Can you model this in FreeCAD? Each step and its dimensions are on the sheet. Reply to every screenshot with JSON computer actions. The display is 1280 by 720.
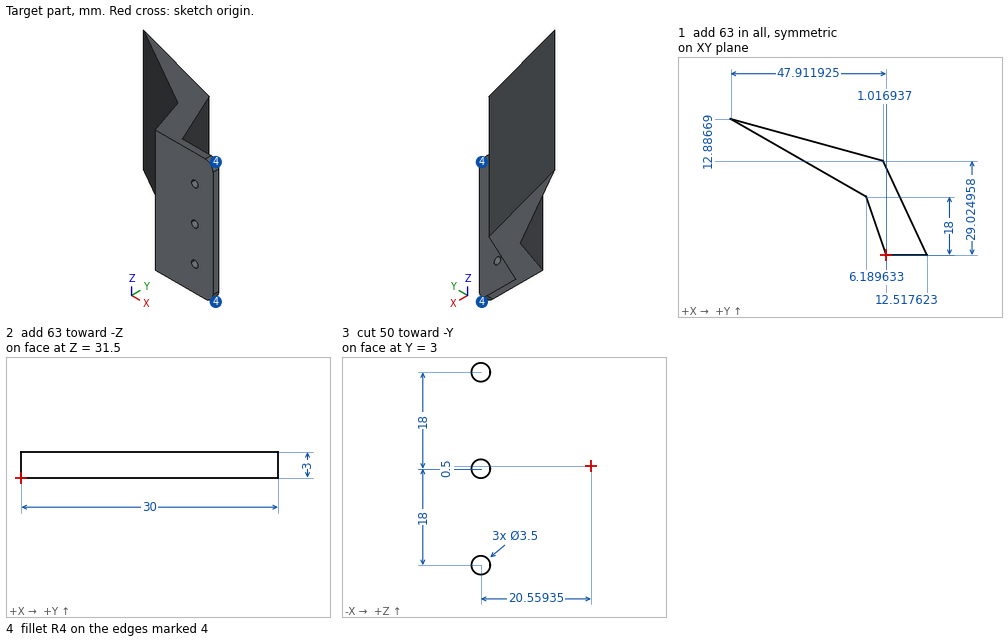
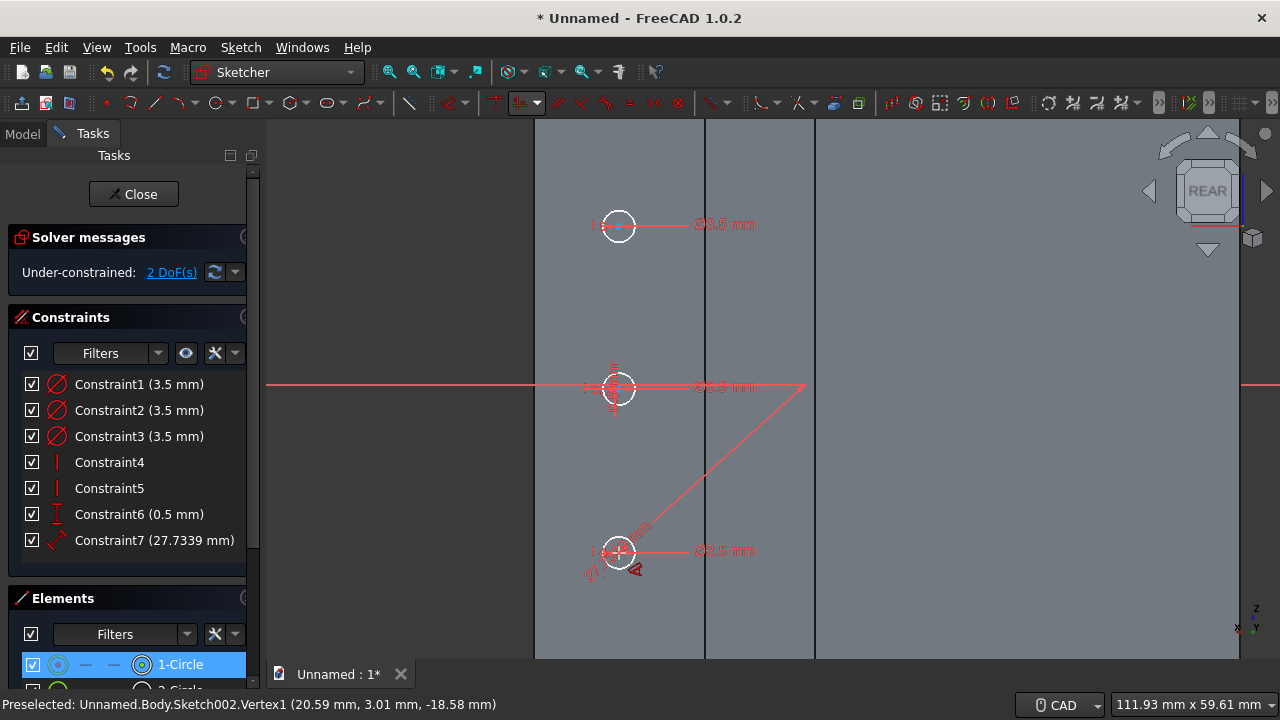
{"action": "left_click", "coordinate": [619, 389]}
{"action": "left_click", "coordinate": [585, 471]}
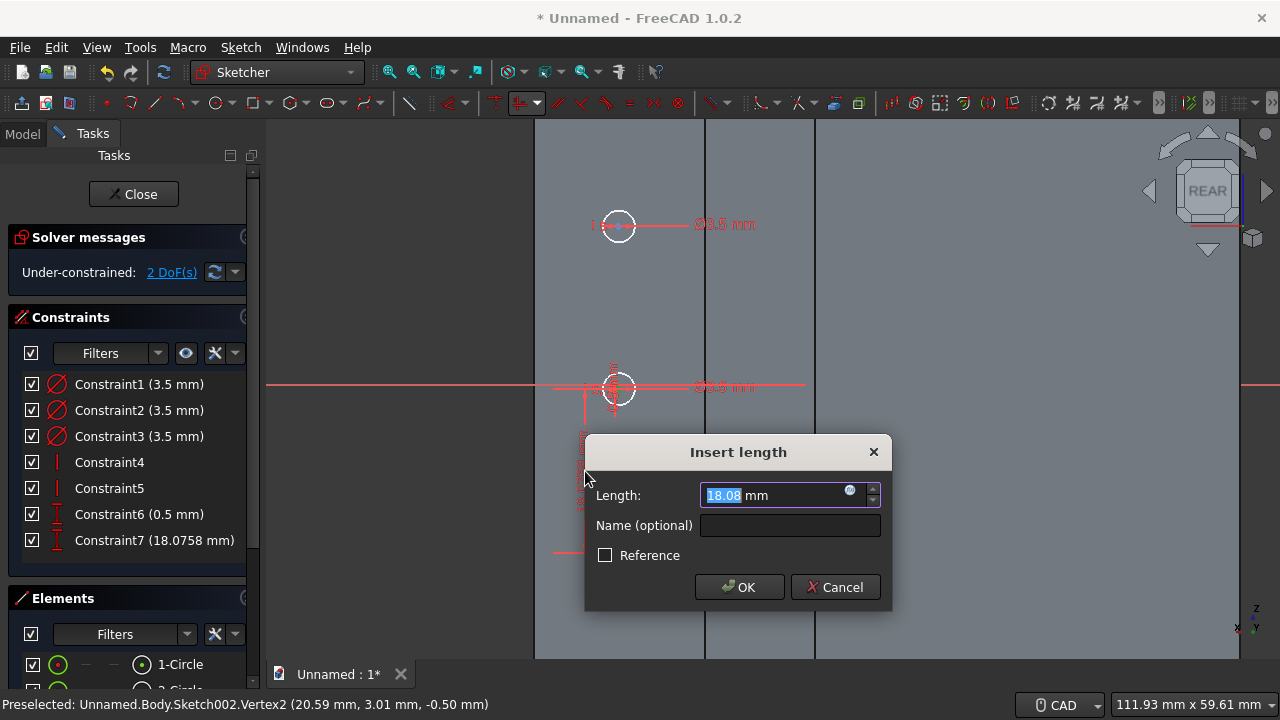
{"action": "type", "text": "18"}
{"action": "key", "text": "Return"}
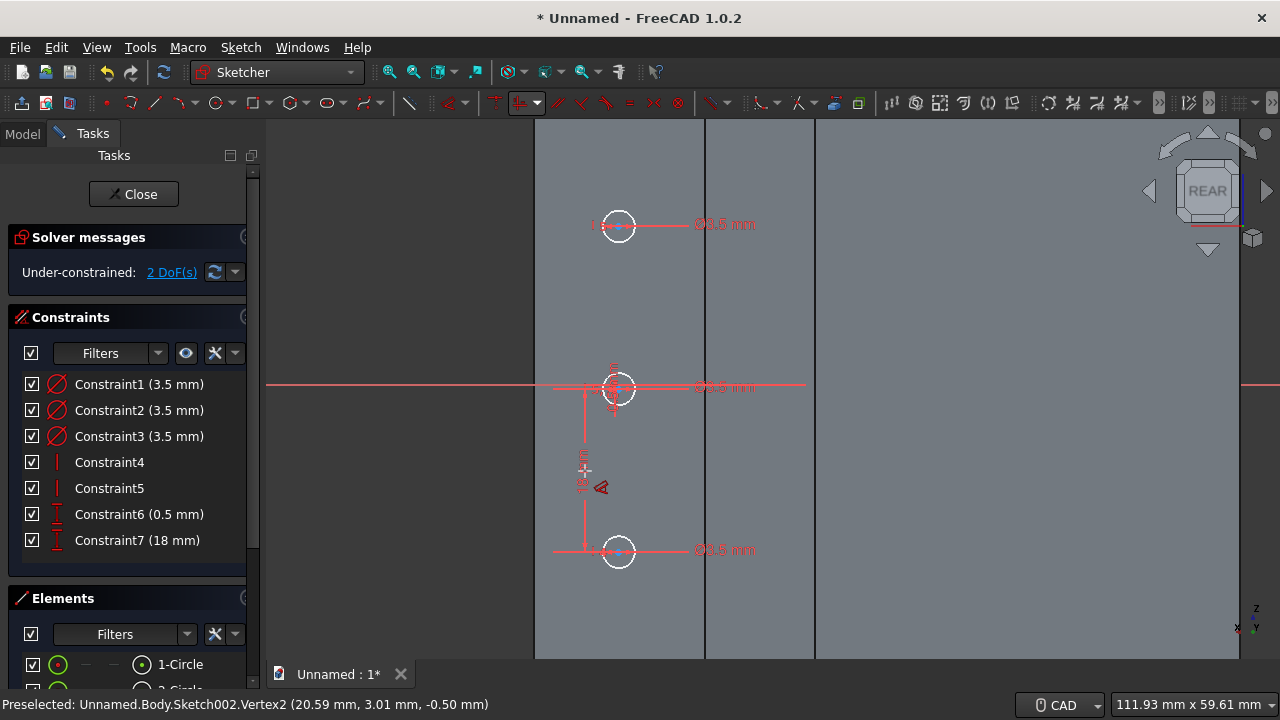
{"action": "left_click", "coordinate": [619, 389]}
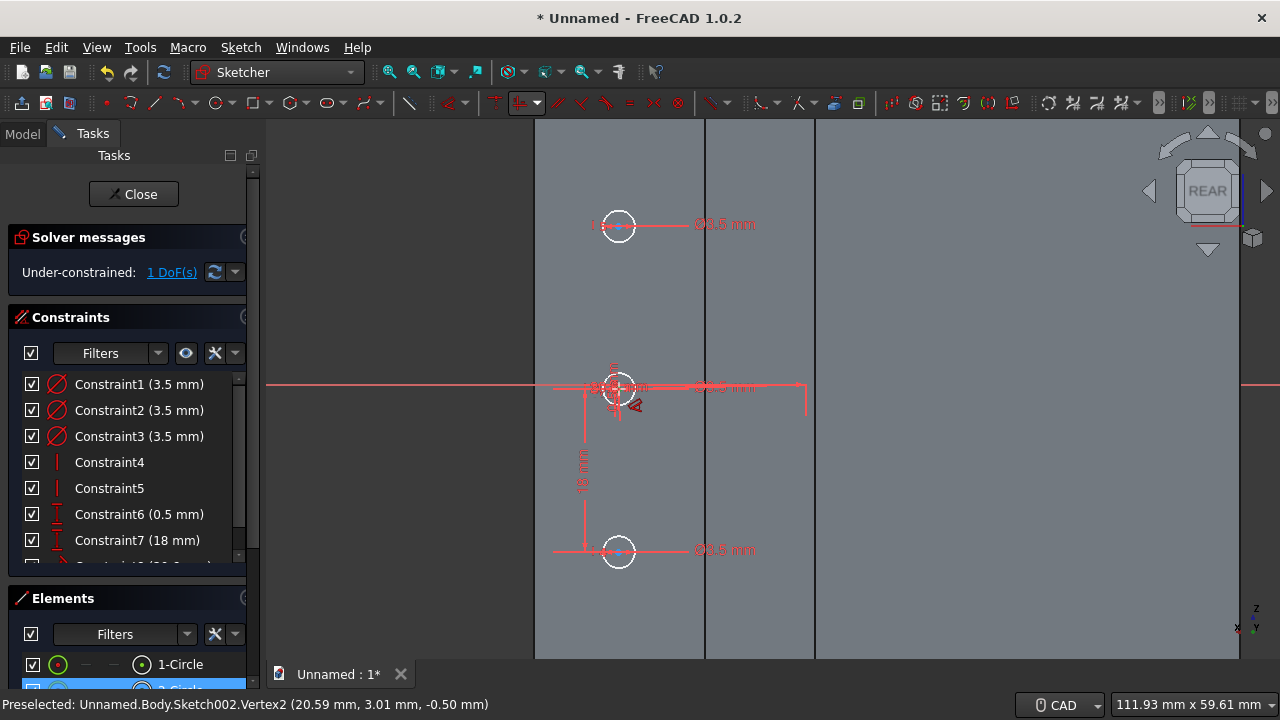
{"action": "left_click", "coordinate": [619, 226]}
{"action": "left_click", "coordinate": [585, 308]}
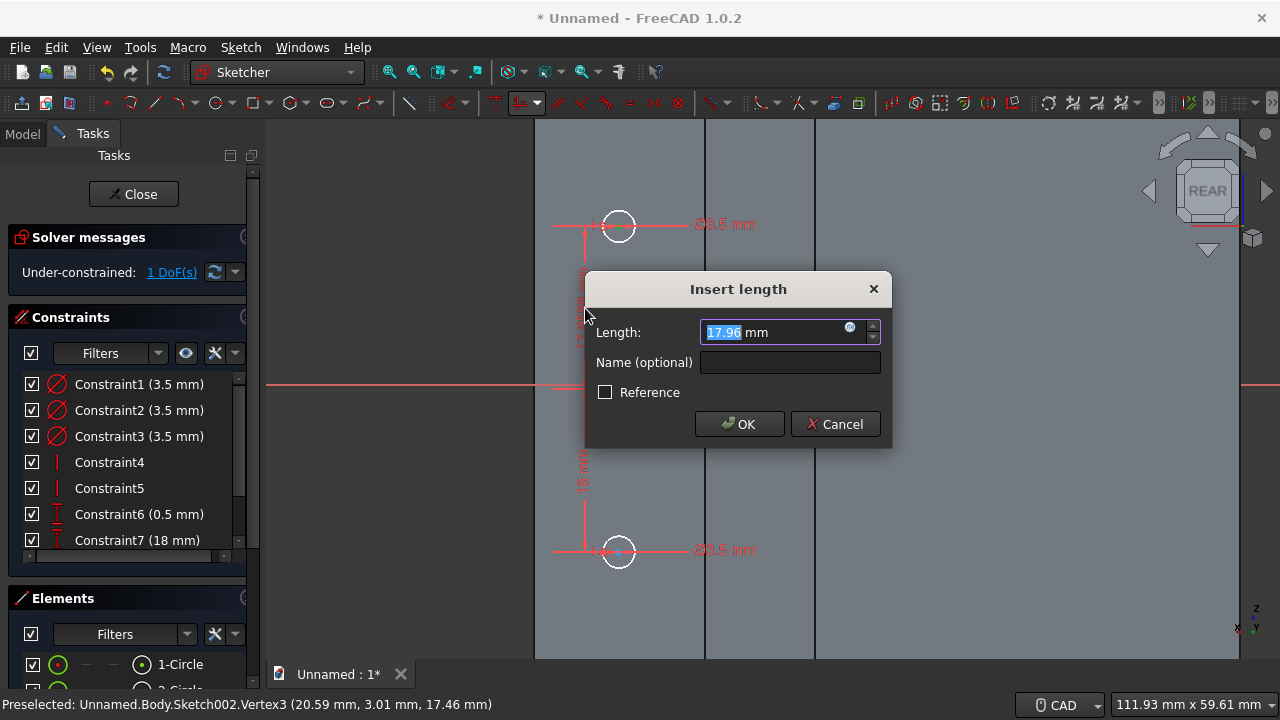
{"action": "type", "text": "18"}
{"action": "key", "text": "Return"}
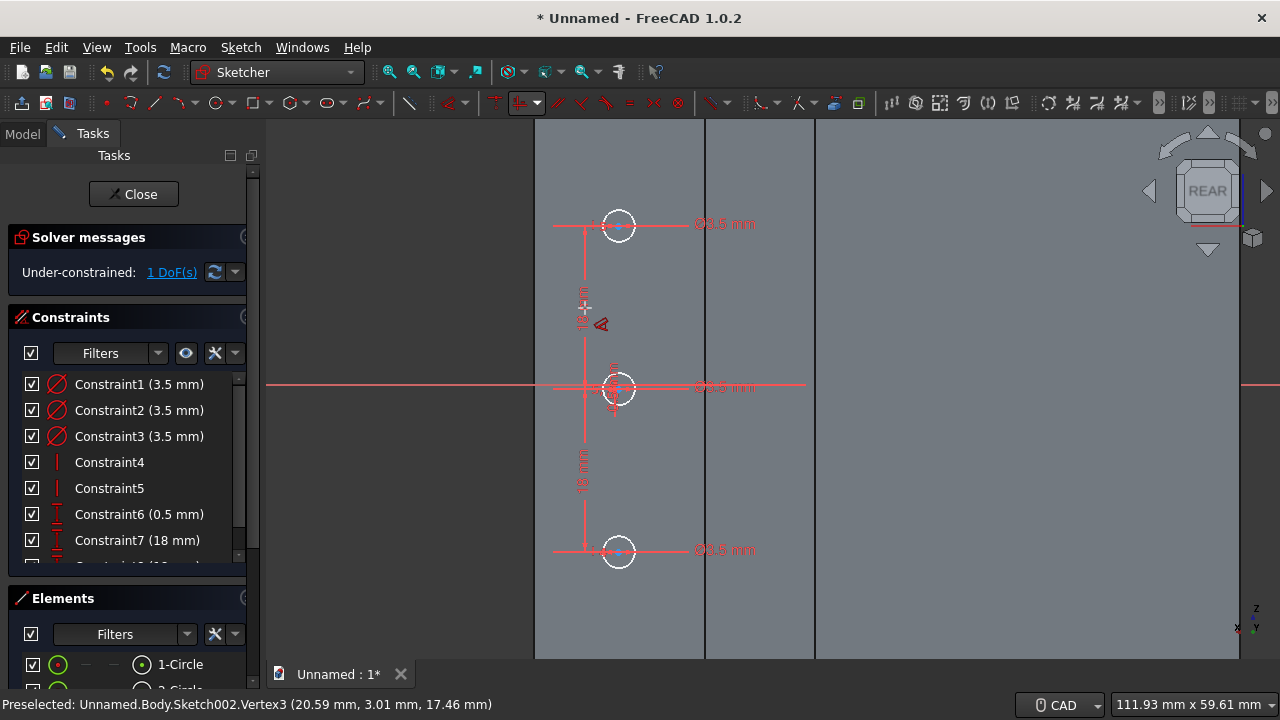
{"action": "left_click", "coordinate": [619, 552]}
{"action": "left_click", "coordinate": [712, 586]}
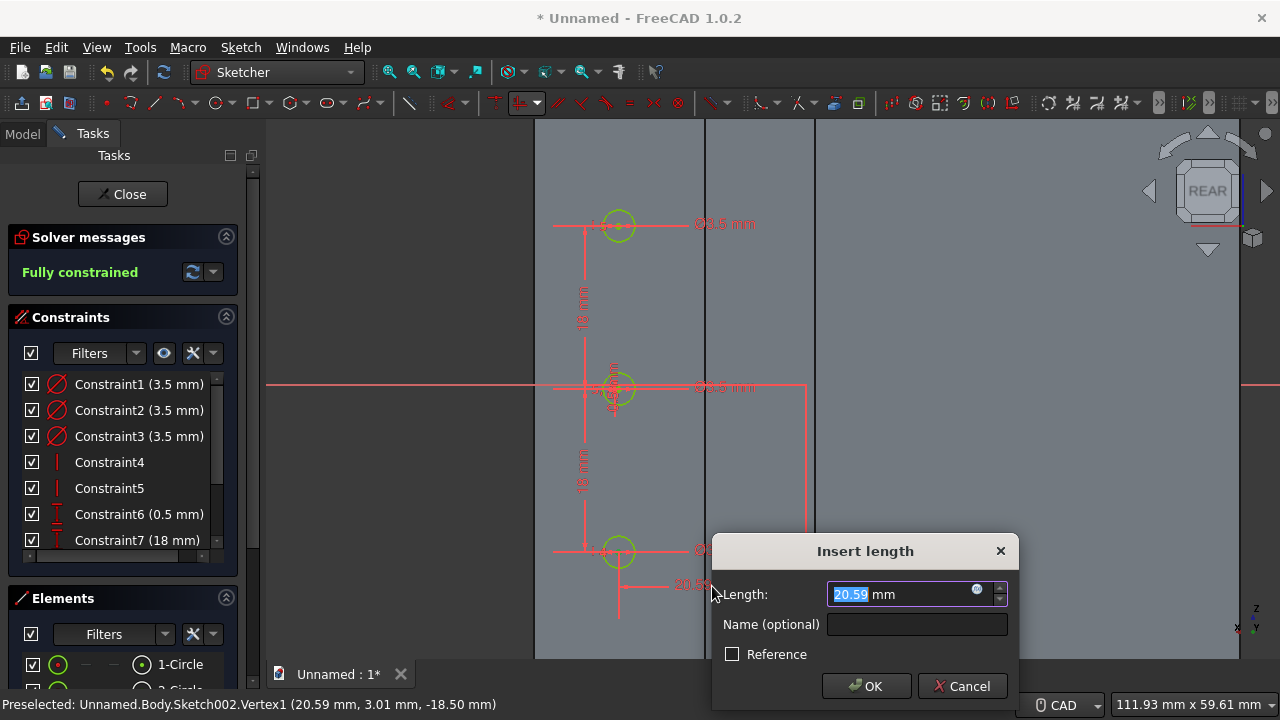
{"action": "type", "text": "20.55935"}
{"action": "key", "text": "Return"}
{"action": "key", "text": "Escape"}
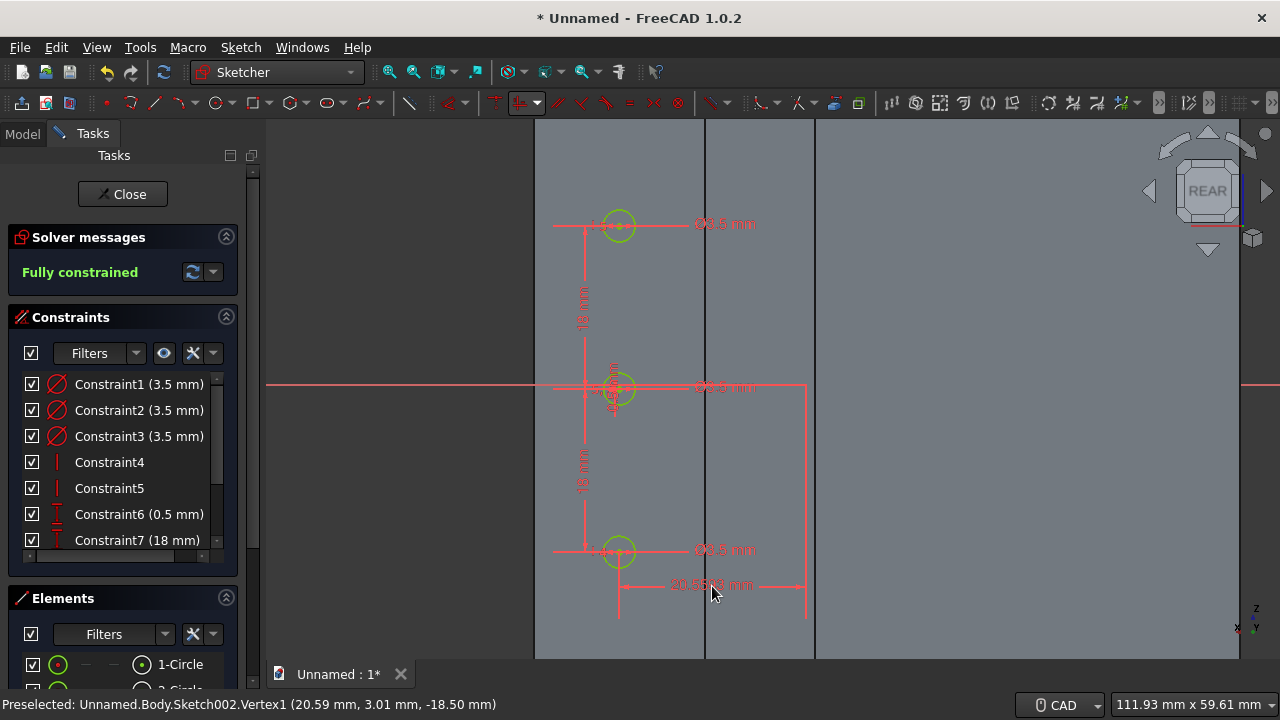
{"action": "left_click", "coordinate": [123, 194]}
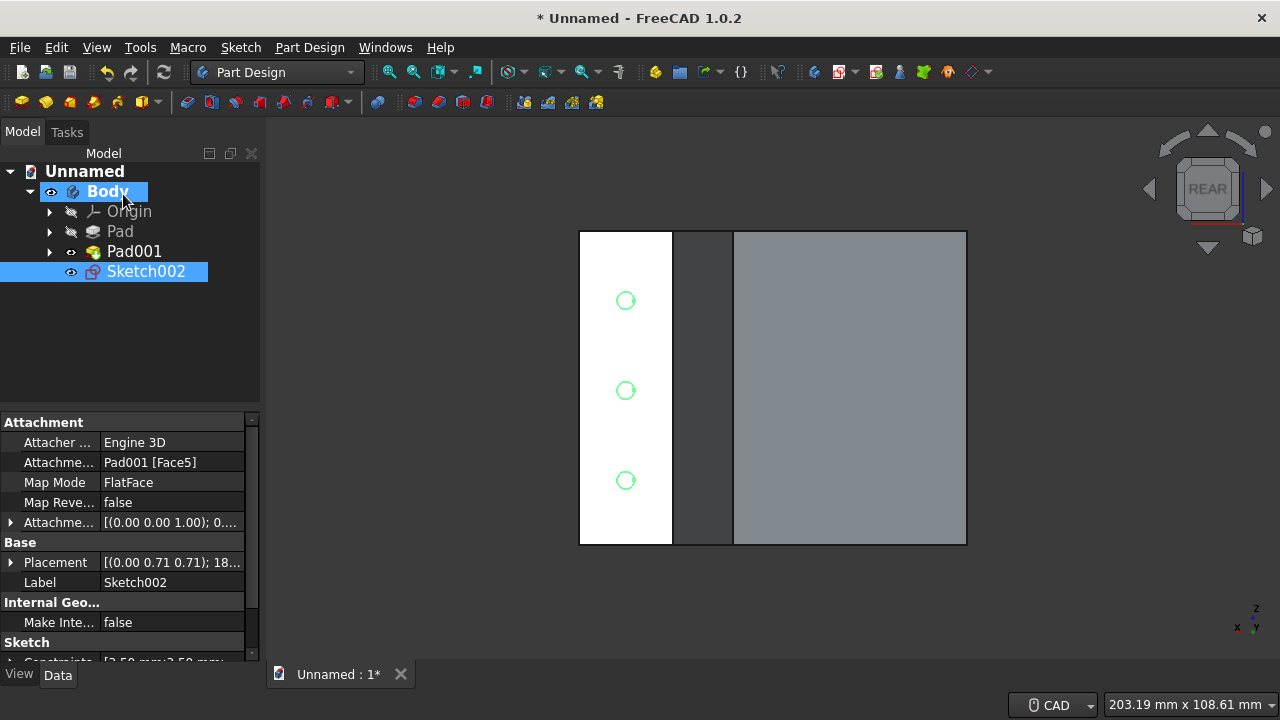
{"action": "left_click", "coordinate": [188, 102]}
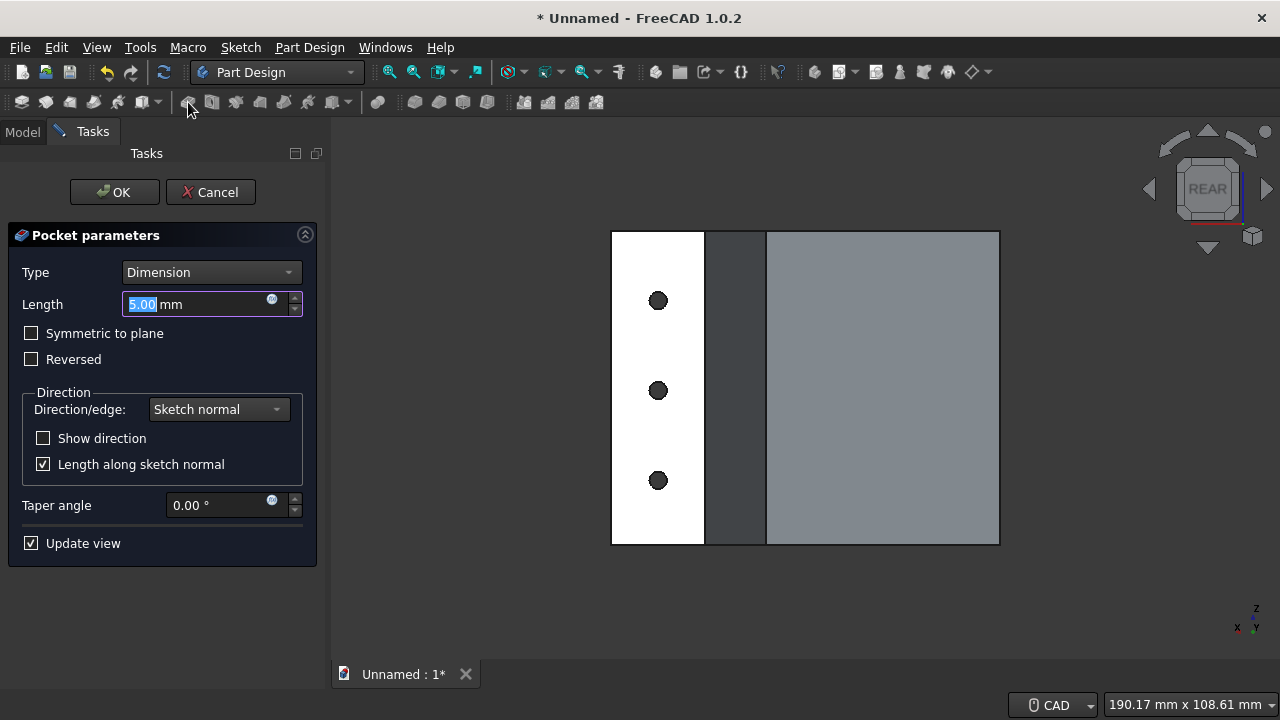
{"action": "type", "text": "50"}
{"action": "key", "text": "Tab"}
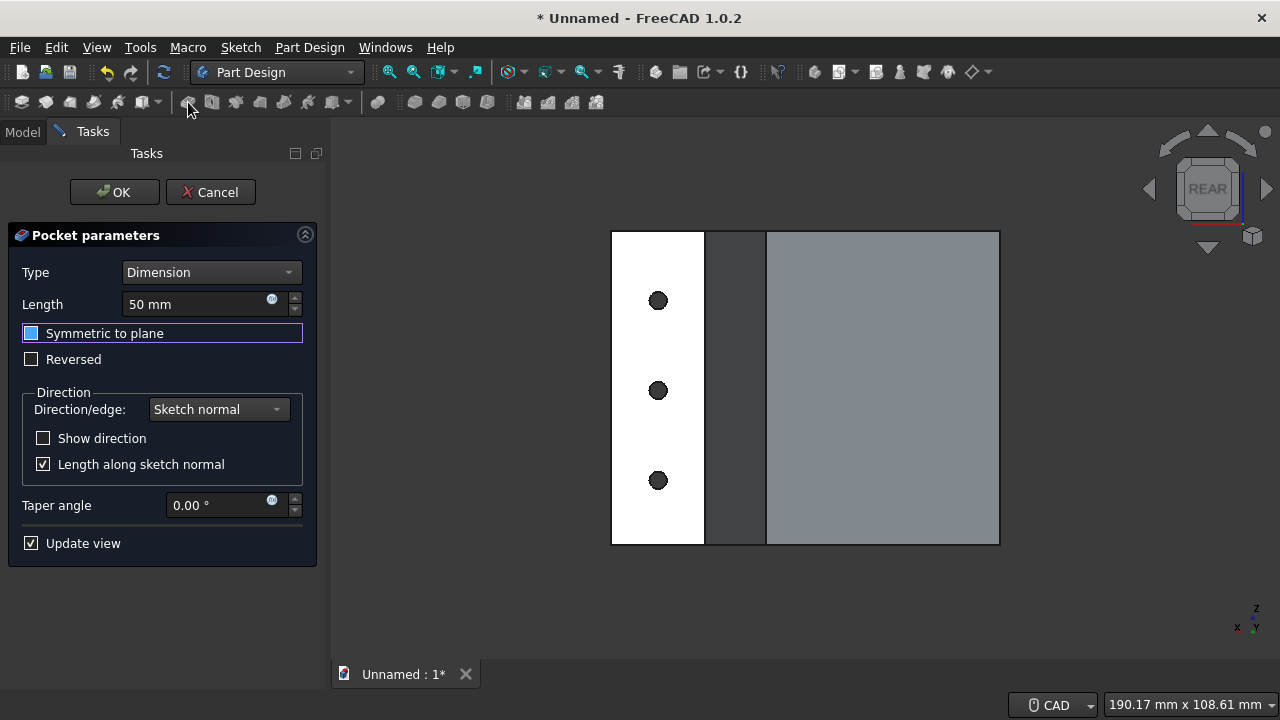
{"action": "left_click", "coordinate": [115, 192]}